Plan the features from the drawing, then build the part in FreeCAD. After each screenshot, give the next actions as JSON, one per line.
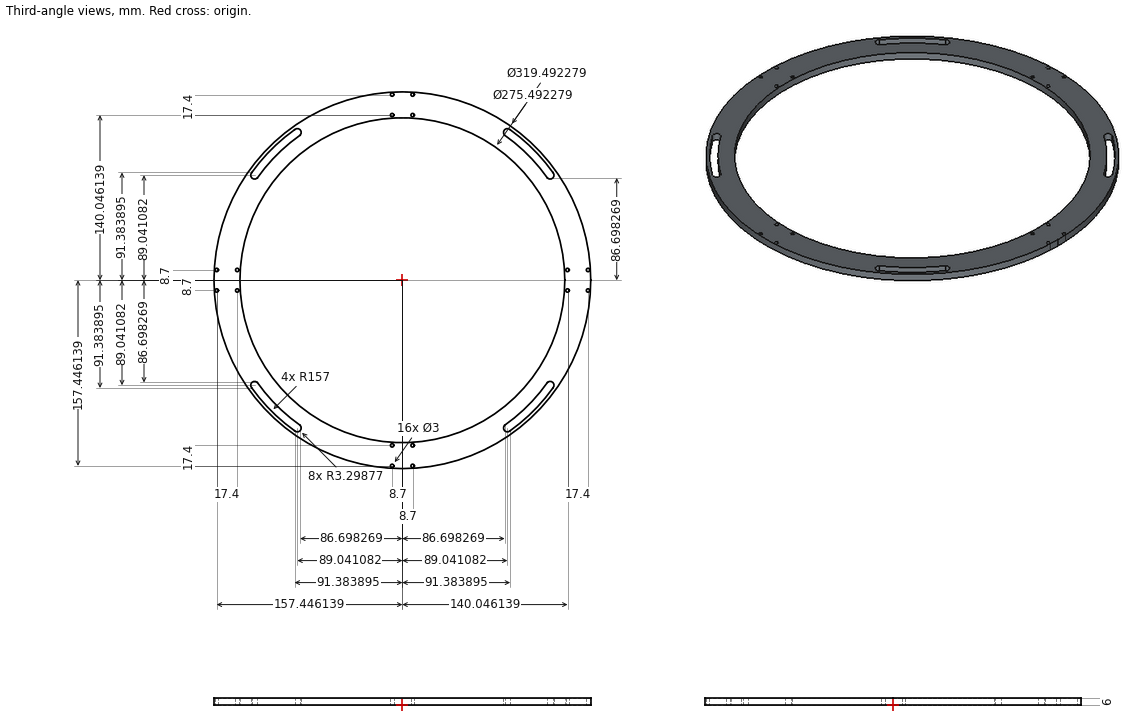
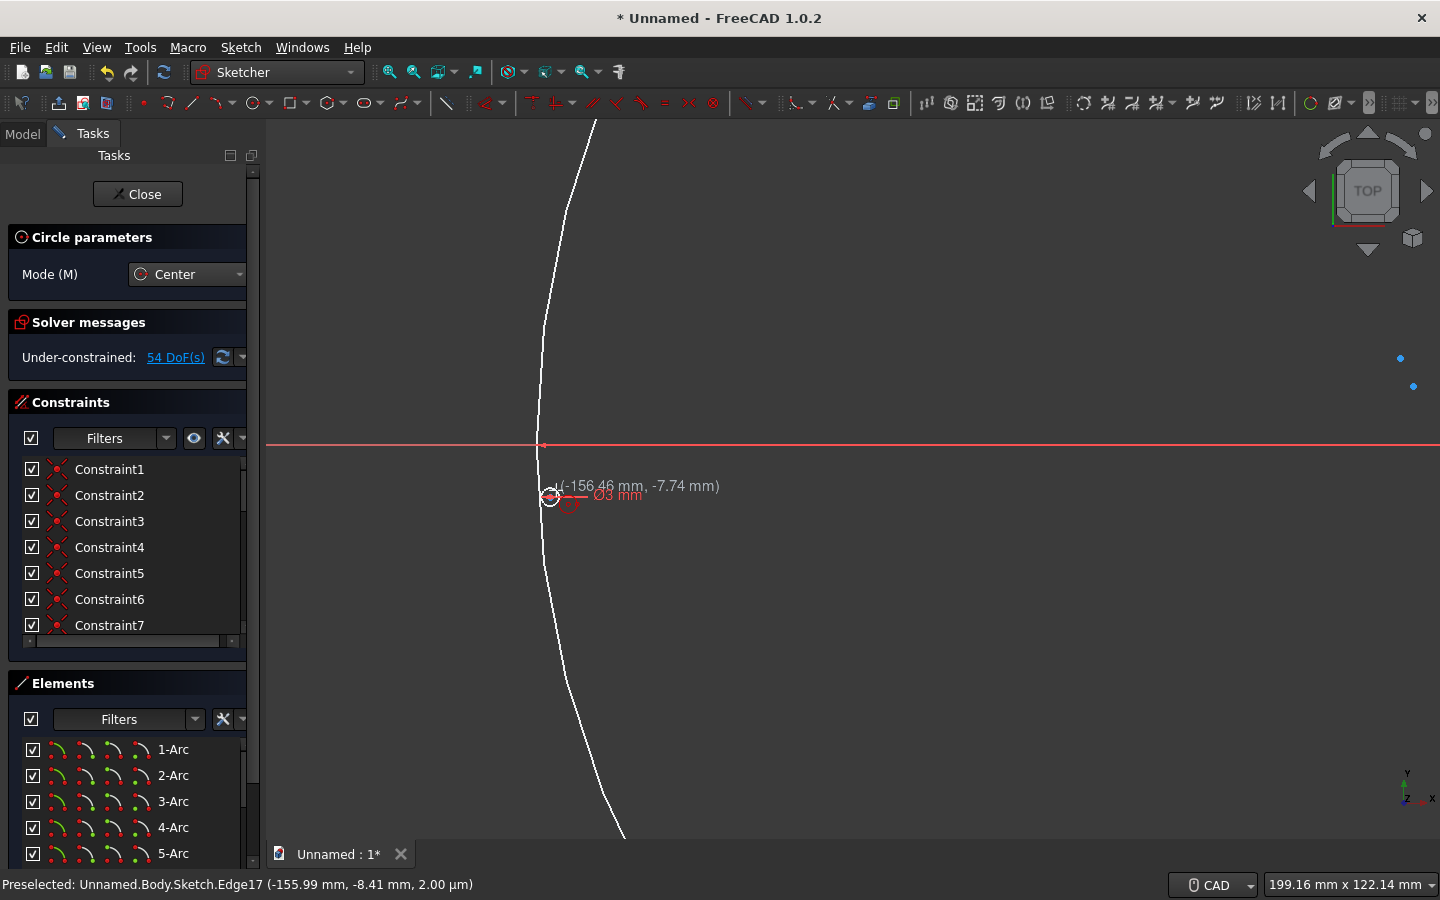
{"action": "scroll", "coordinate": [653, 497], "scroll_direction": "up", "scroll_amount": 5}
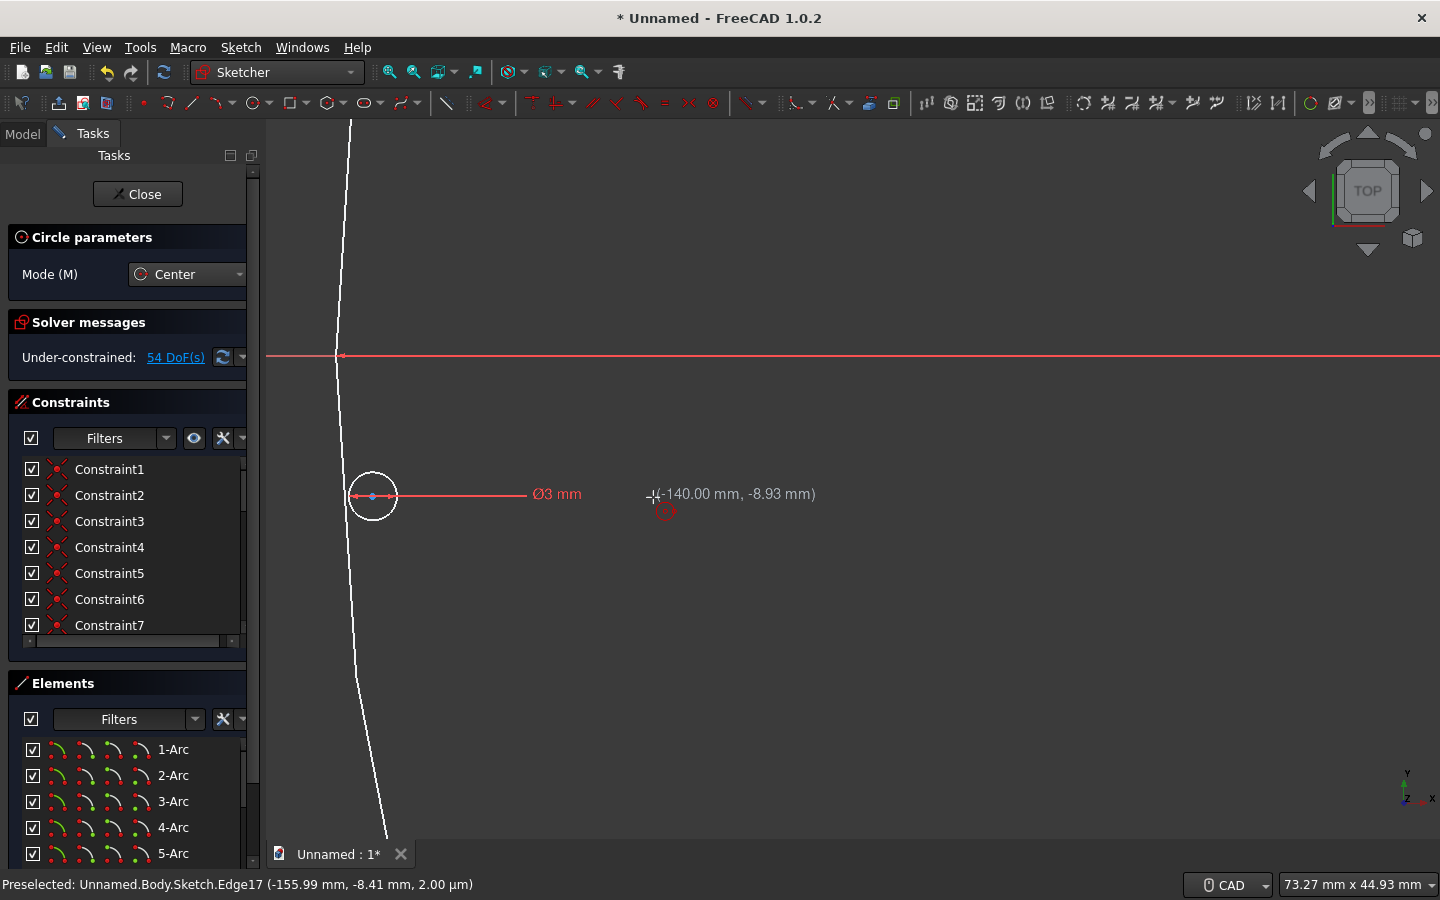
{"action": "scroll", "coordinate": [574, 491], "scroll_direction": "down", "scroll_amount": 12}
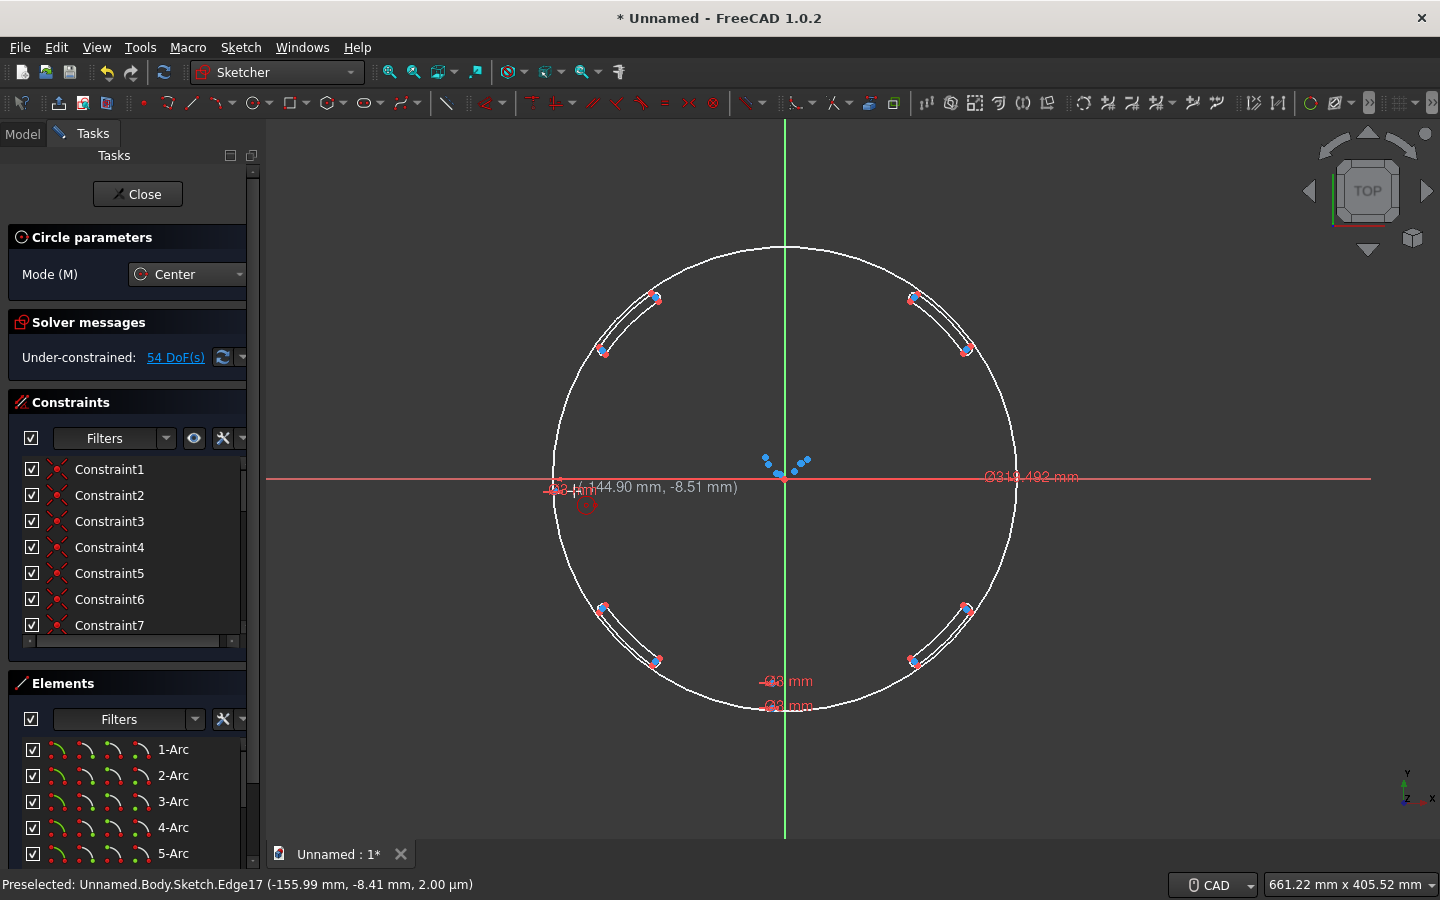
{"action": "scroll", "coordinate": [581, 492], "scroll_direction": "up", "scroll_amount": 2}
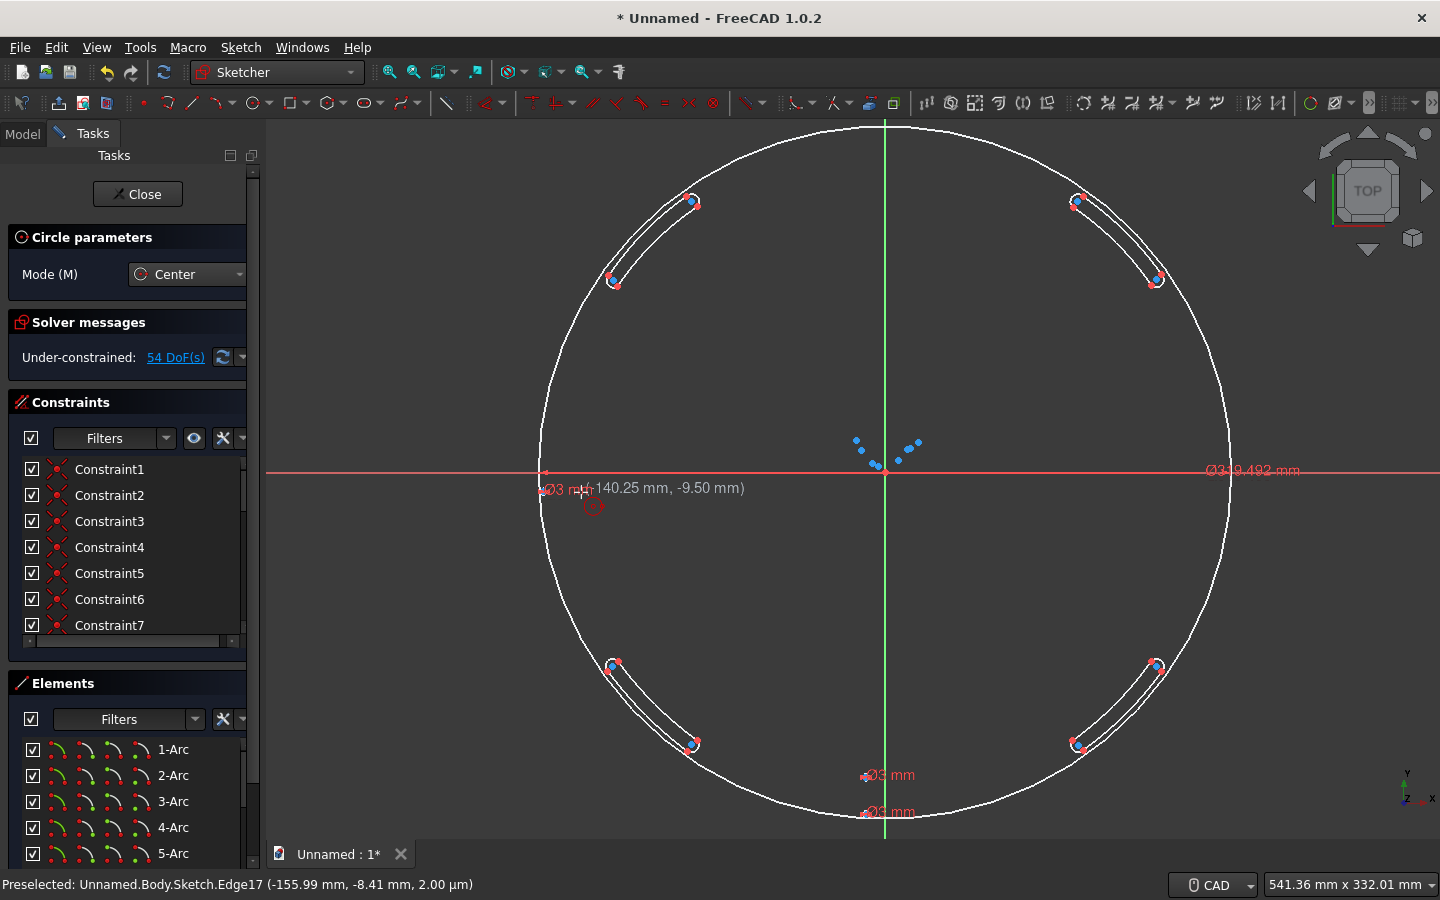
{"action": "left_click", "coordinate": [581, 492]}
{"action": "mouse_move", "coordinate": [584, 489]}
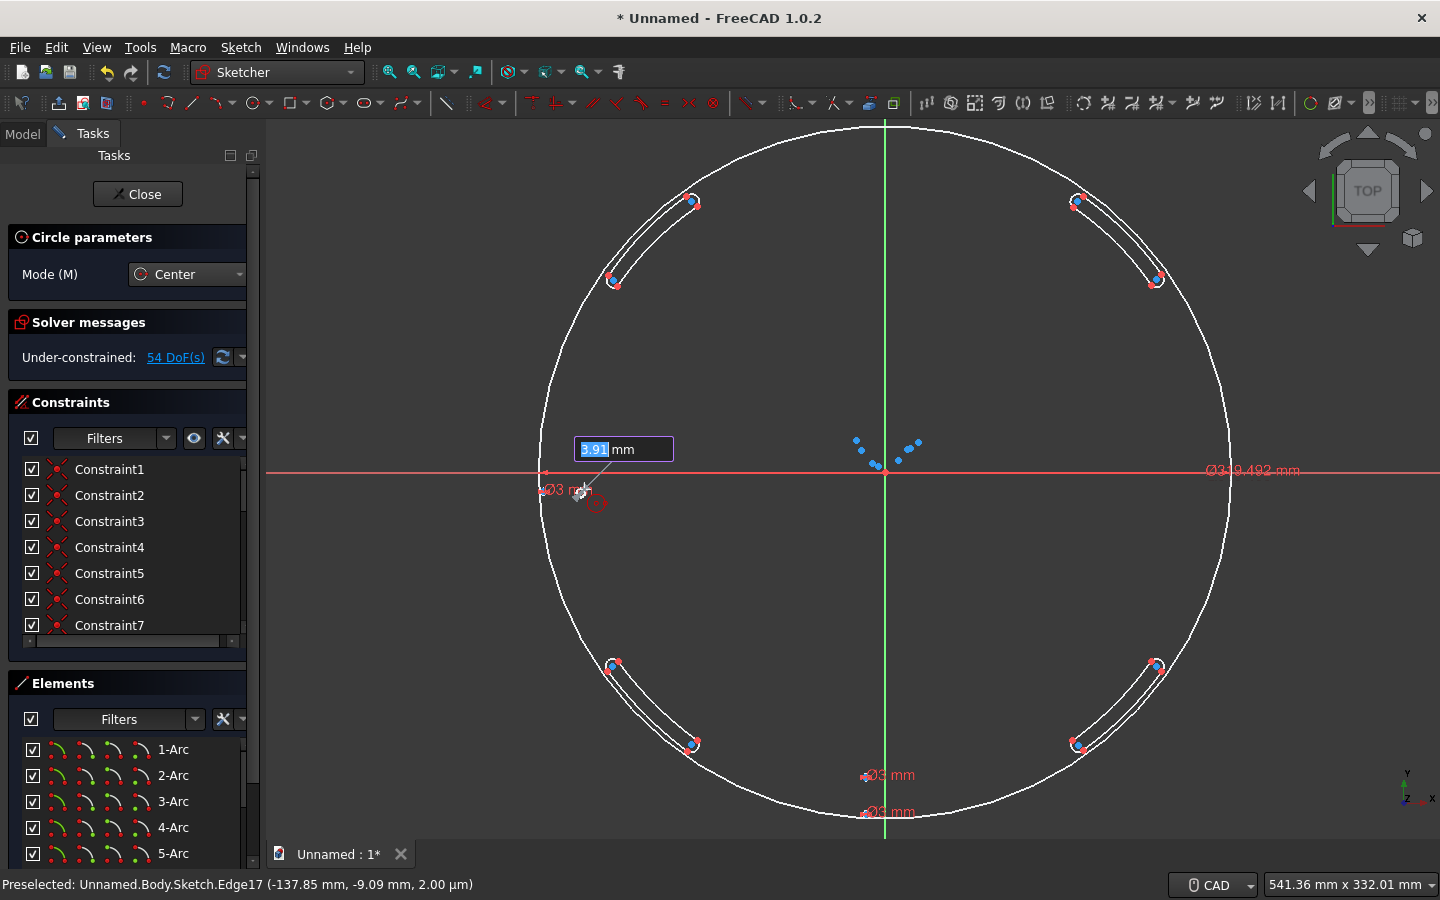
{"action": "type", "text": "3"}
{"action": "key", "text": "Return"}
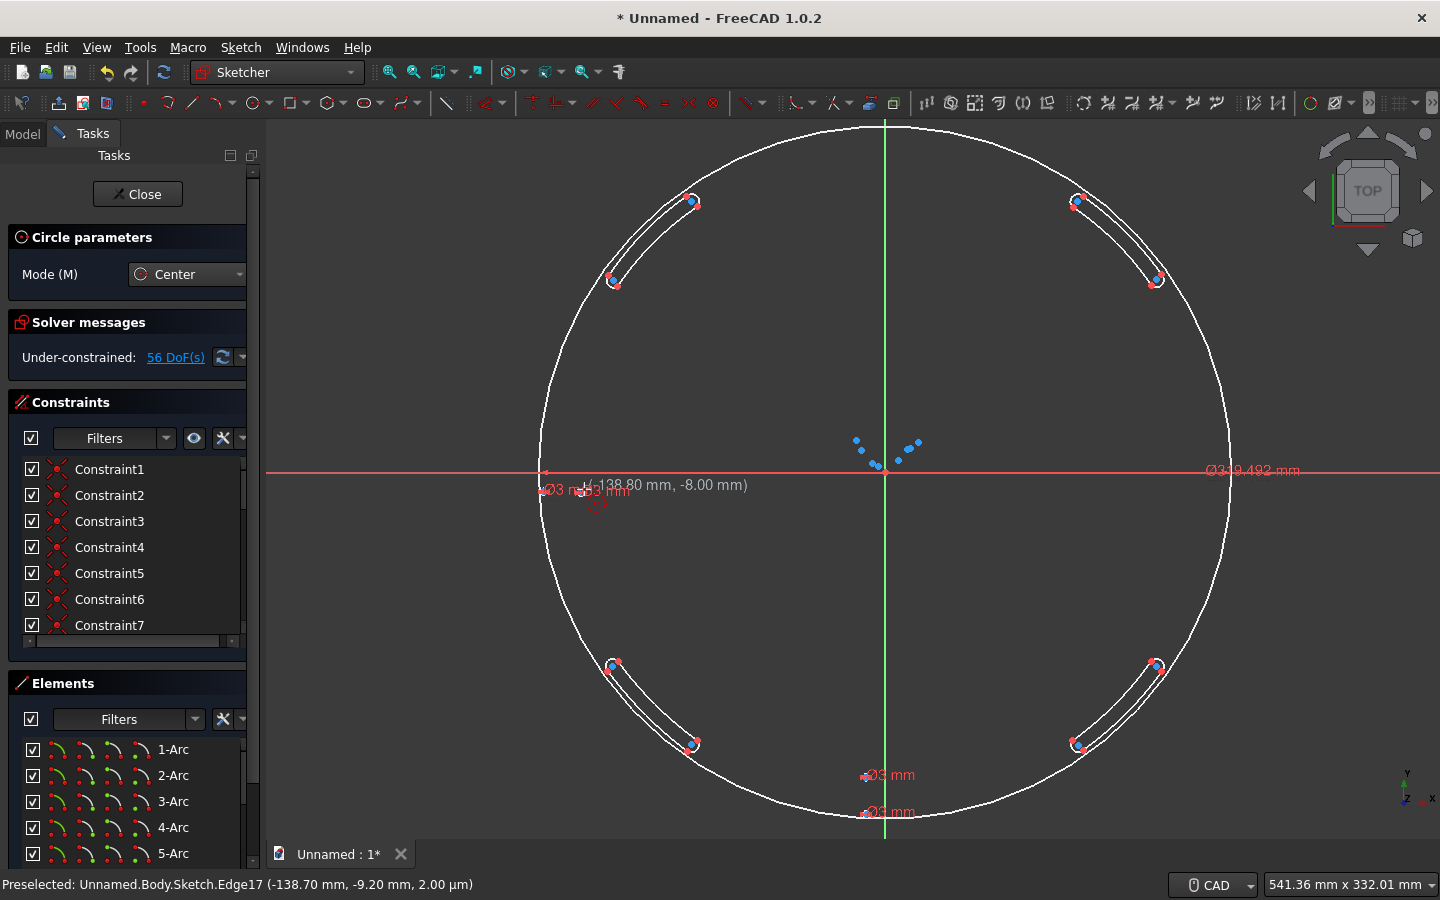
{"action": "scroll", "coordinate": [580, 492], "scroll_direction": "down", "scroll_amount": 2}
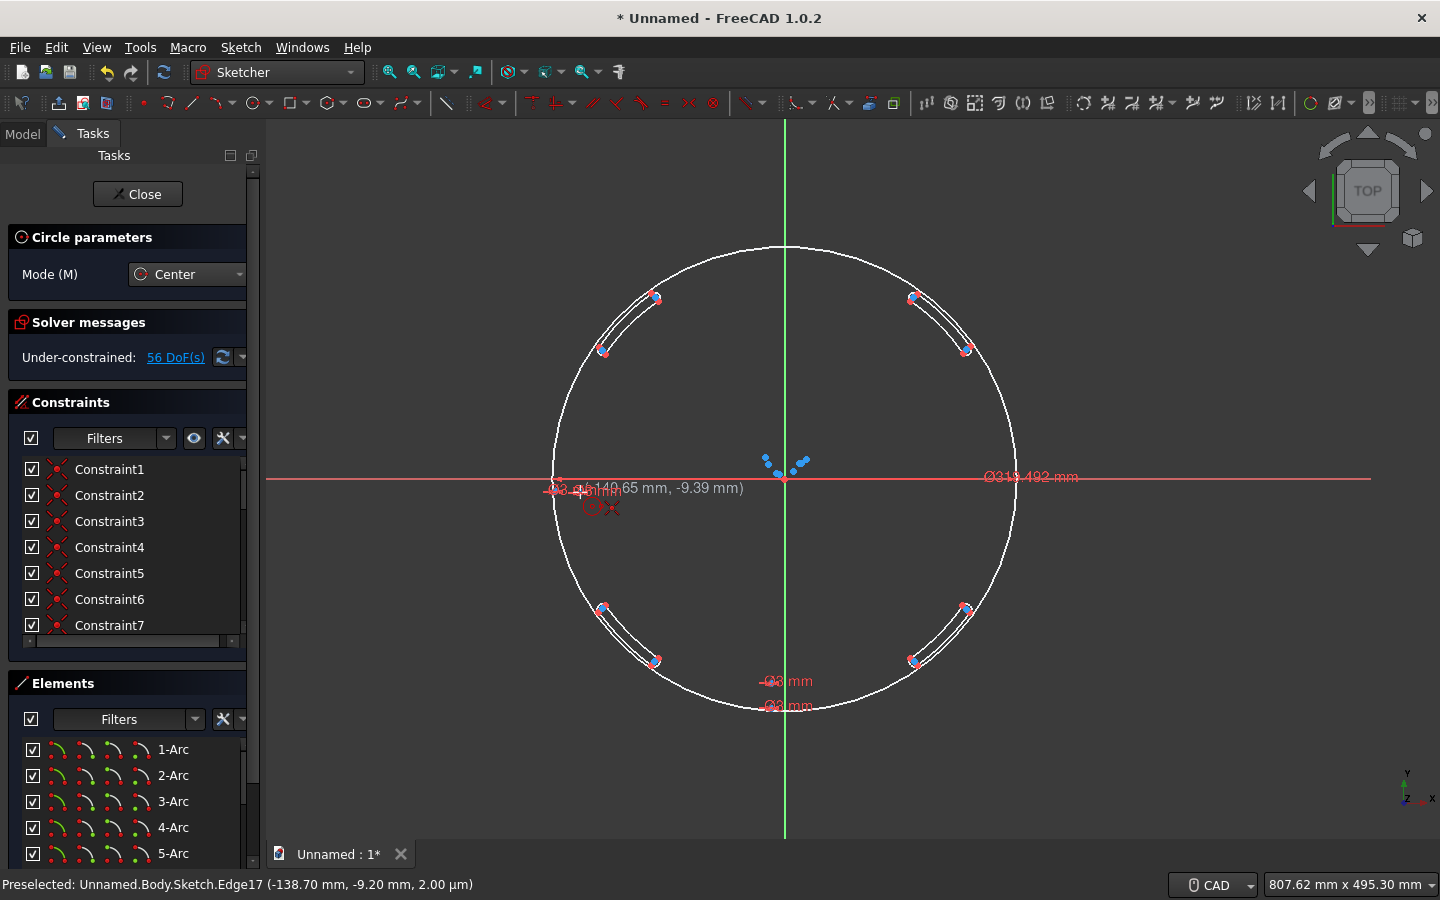
{"action": "scroll", "coordinate": [797, 708], "scroll_direction": "up", "scroll_amount": 12}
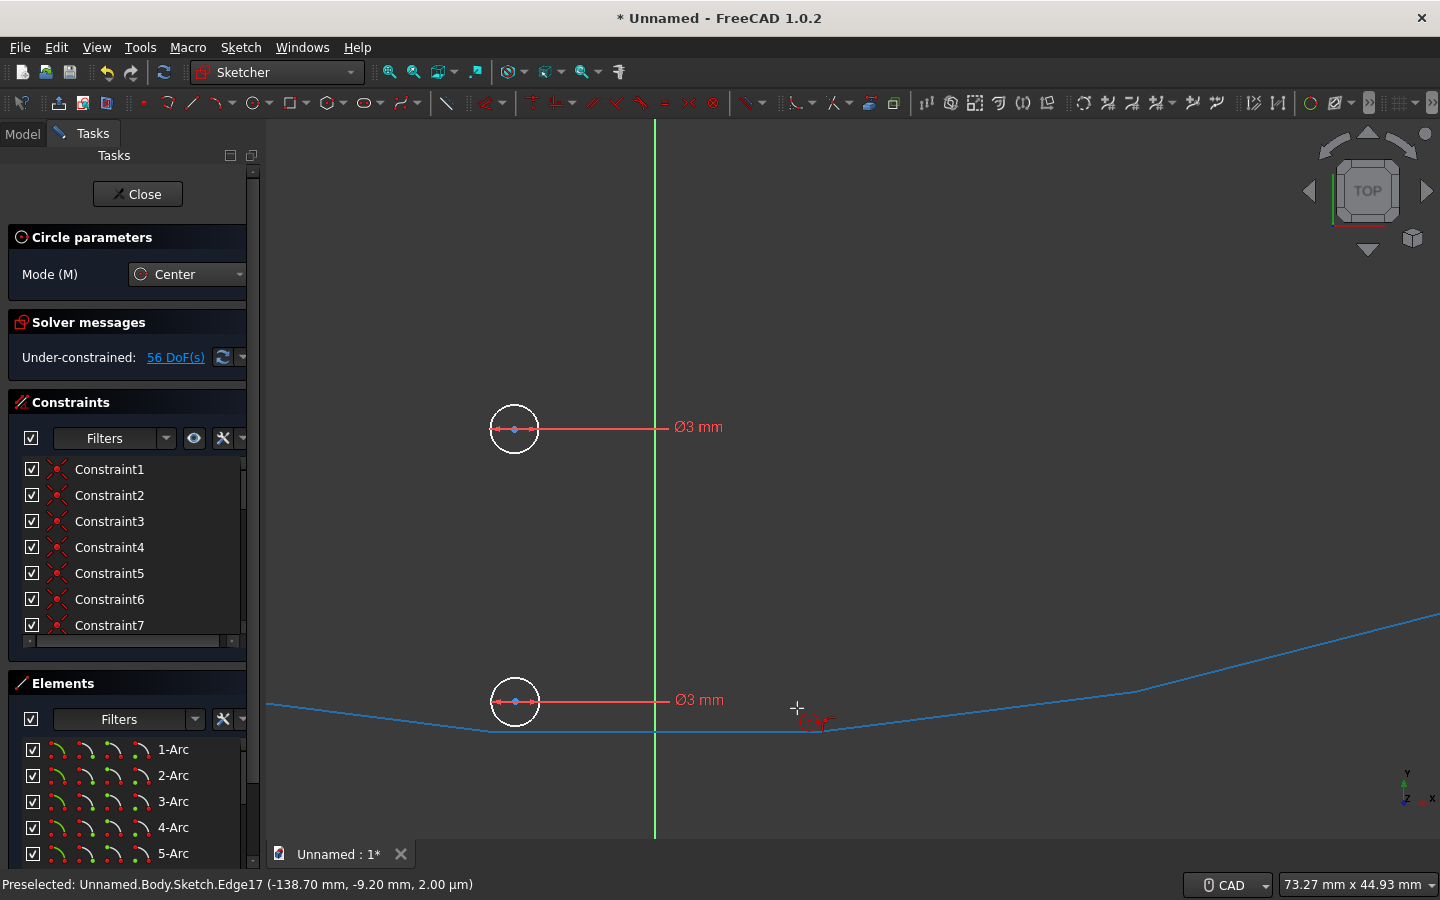
{"action": "left_click", "coordinate": [794, 701]}